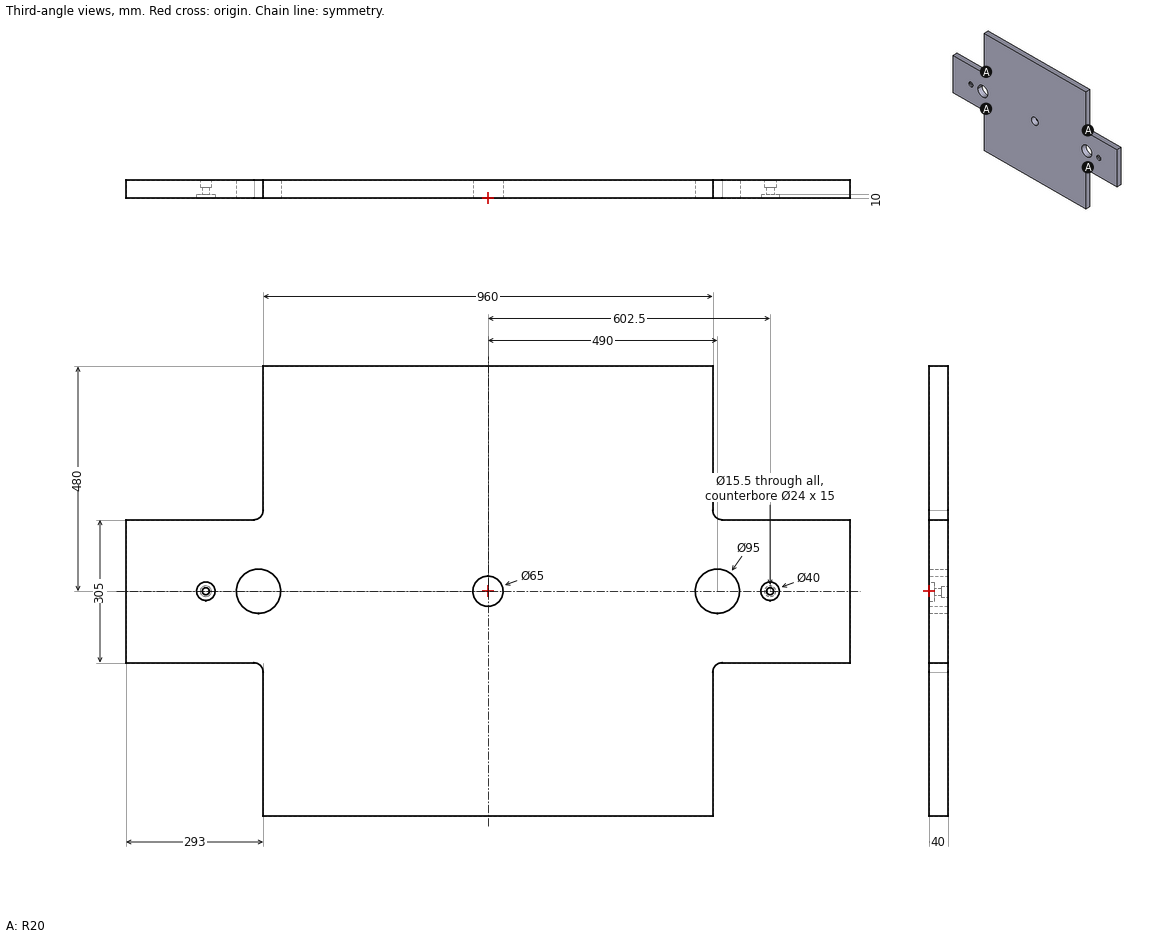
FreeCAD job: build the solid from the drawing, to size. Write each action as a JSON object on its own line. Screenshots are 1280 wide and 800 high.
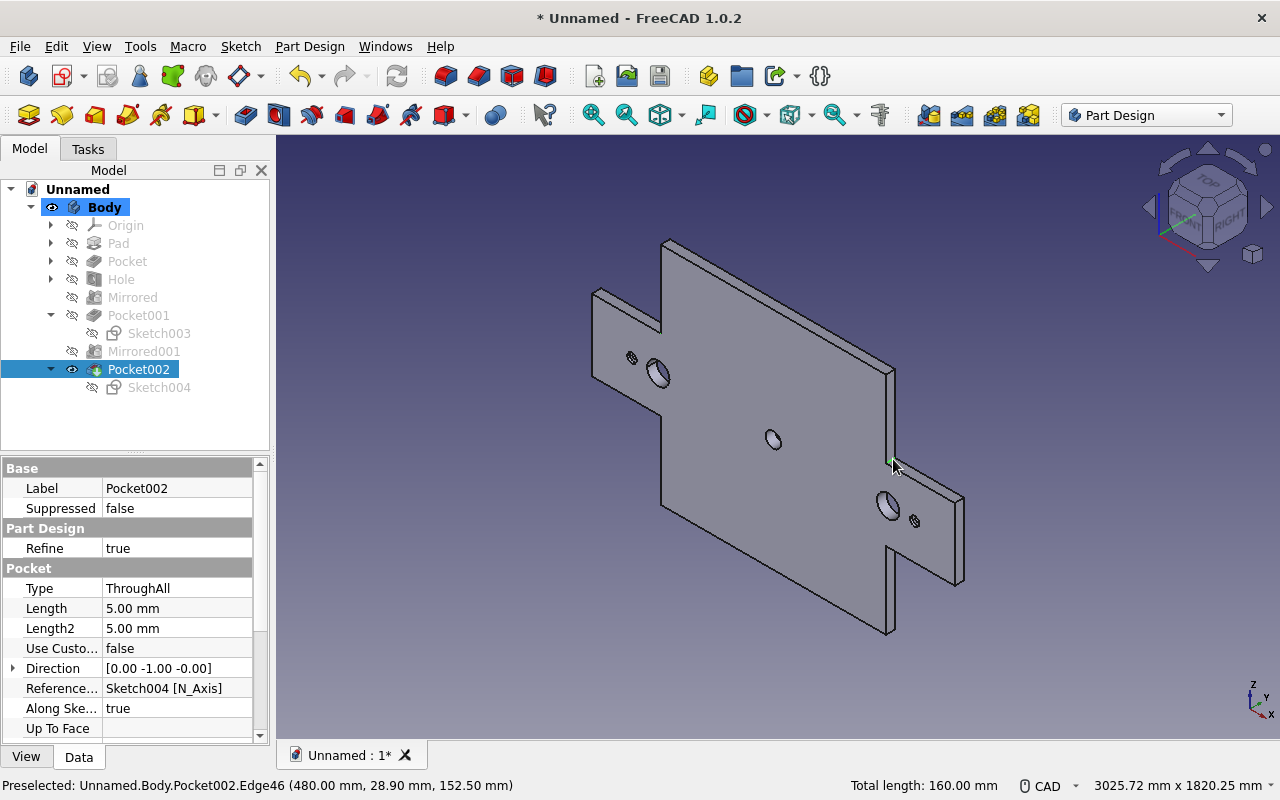
{"action": "left_click", "coordinate": [446, 76]}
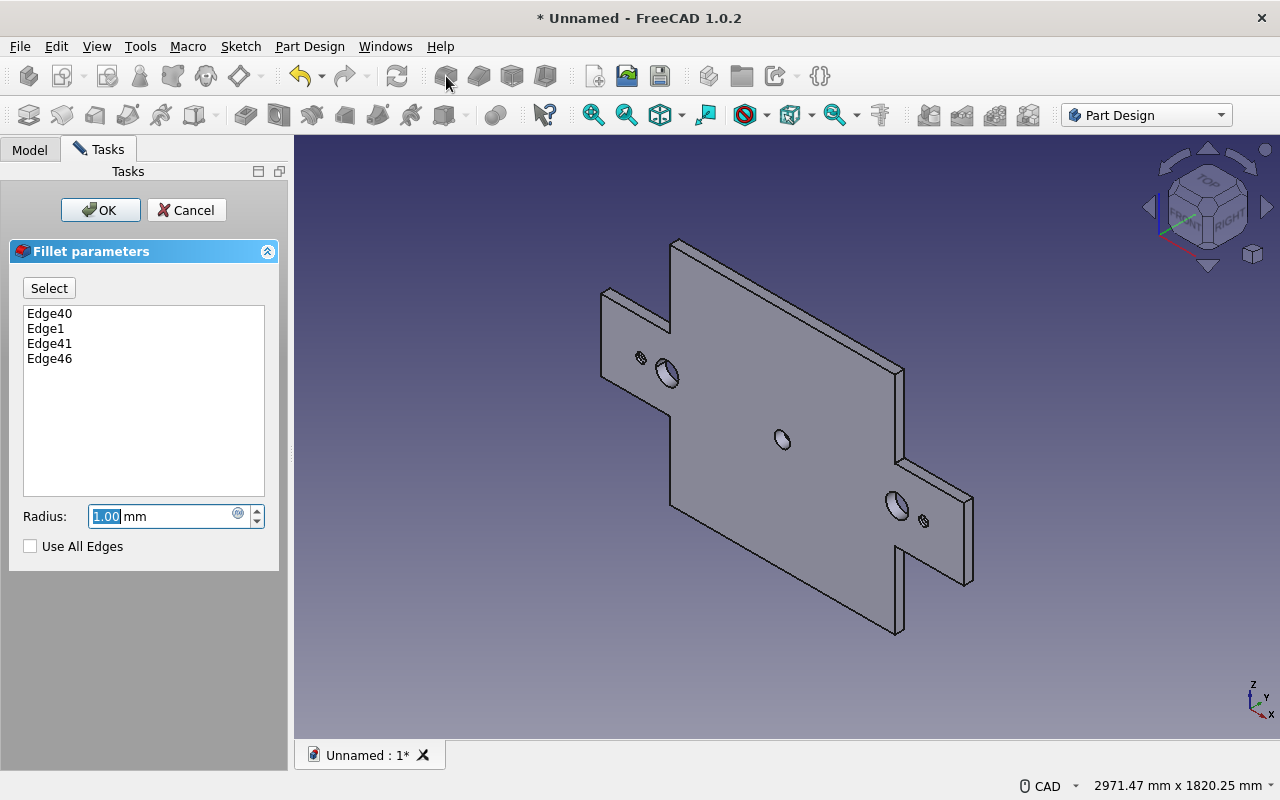
{"action": "type", "text": "20"}
{"action": "key", "text": "Tab"}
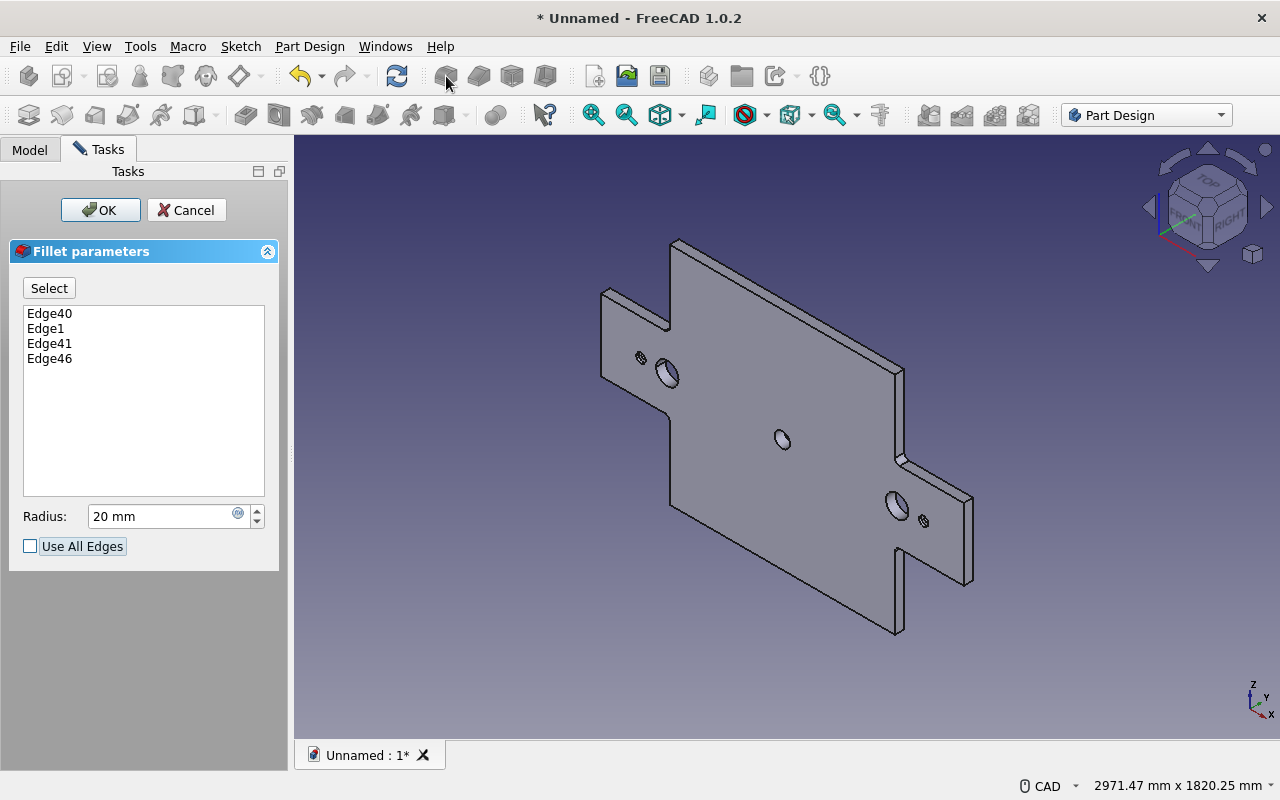
{"action": "left_click", "coordinate": [101, 210]}